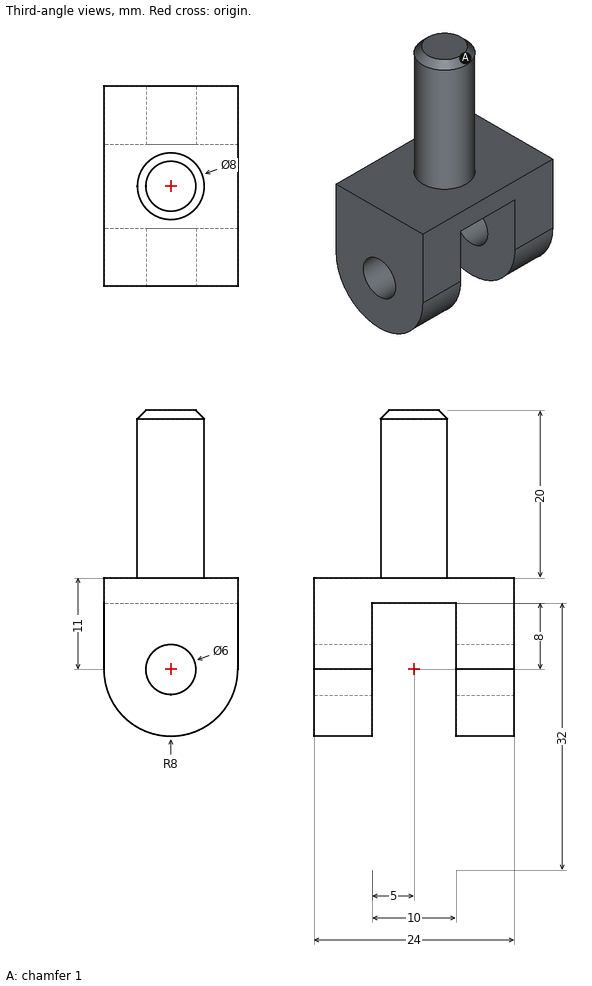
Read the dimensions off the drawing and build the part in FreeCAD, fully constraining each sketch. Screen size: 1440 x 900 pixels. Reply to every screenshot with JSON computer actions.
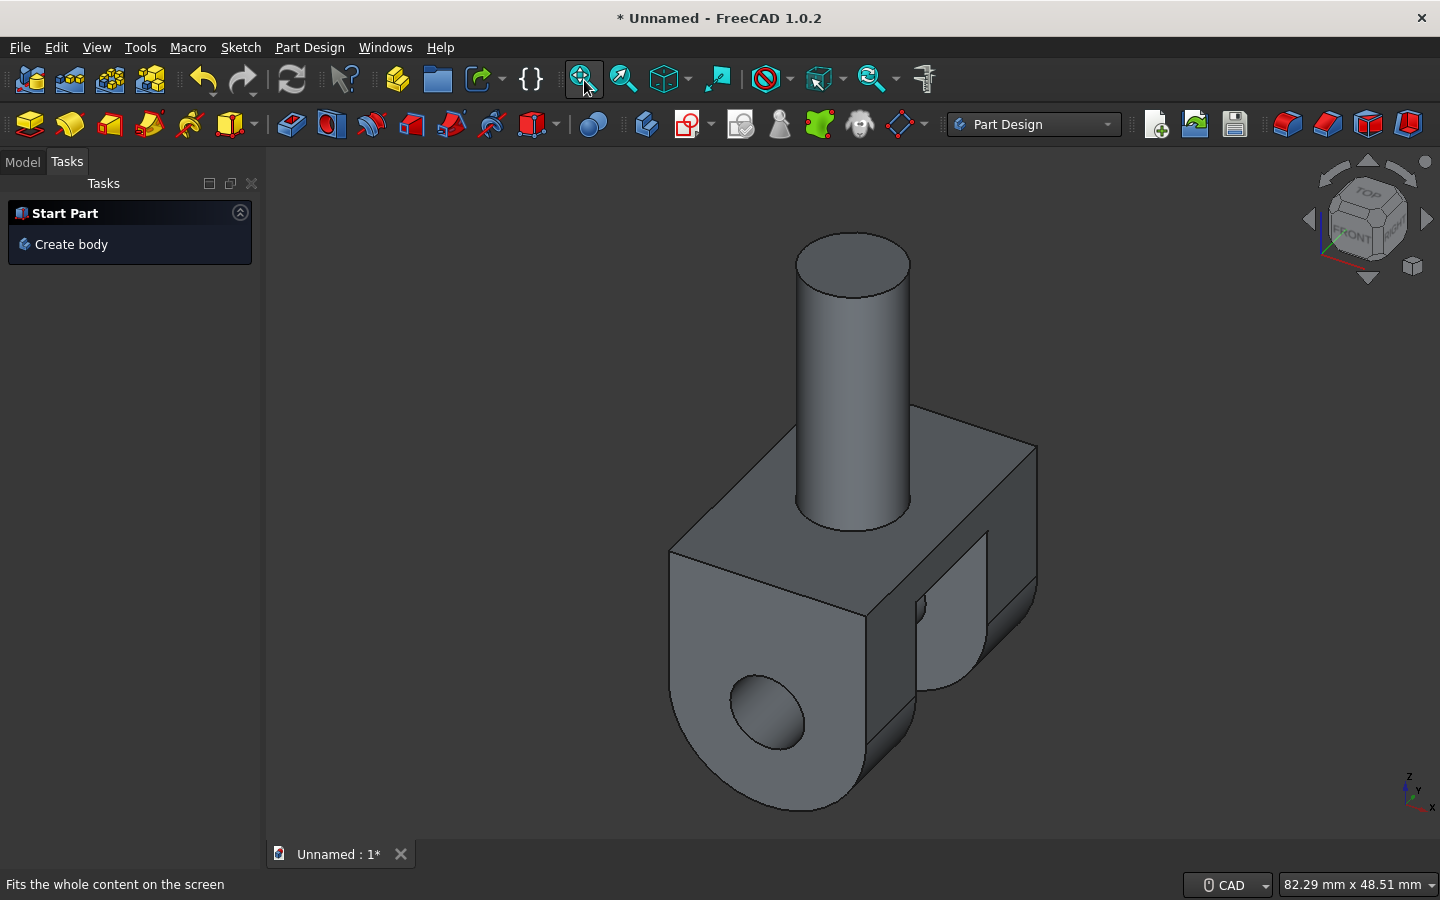
{"action": "left_click", "coordinate": [902, 280]}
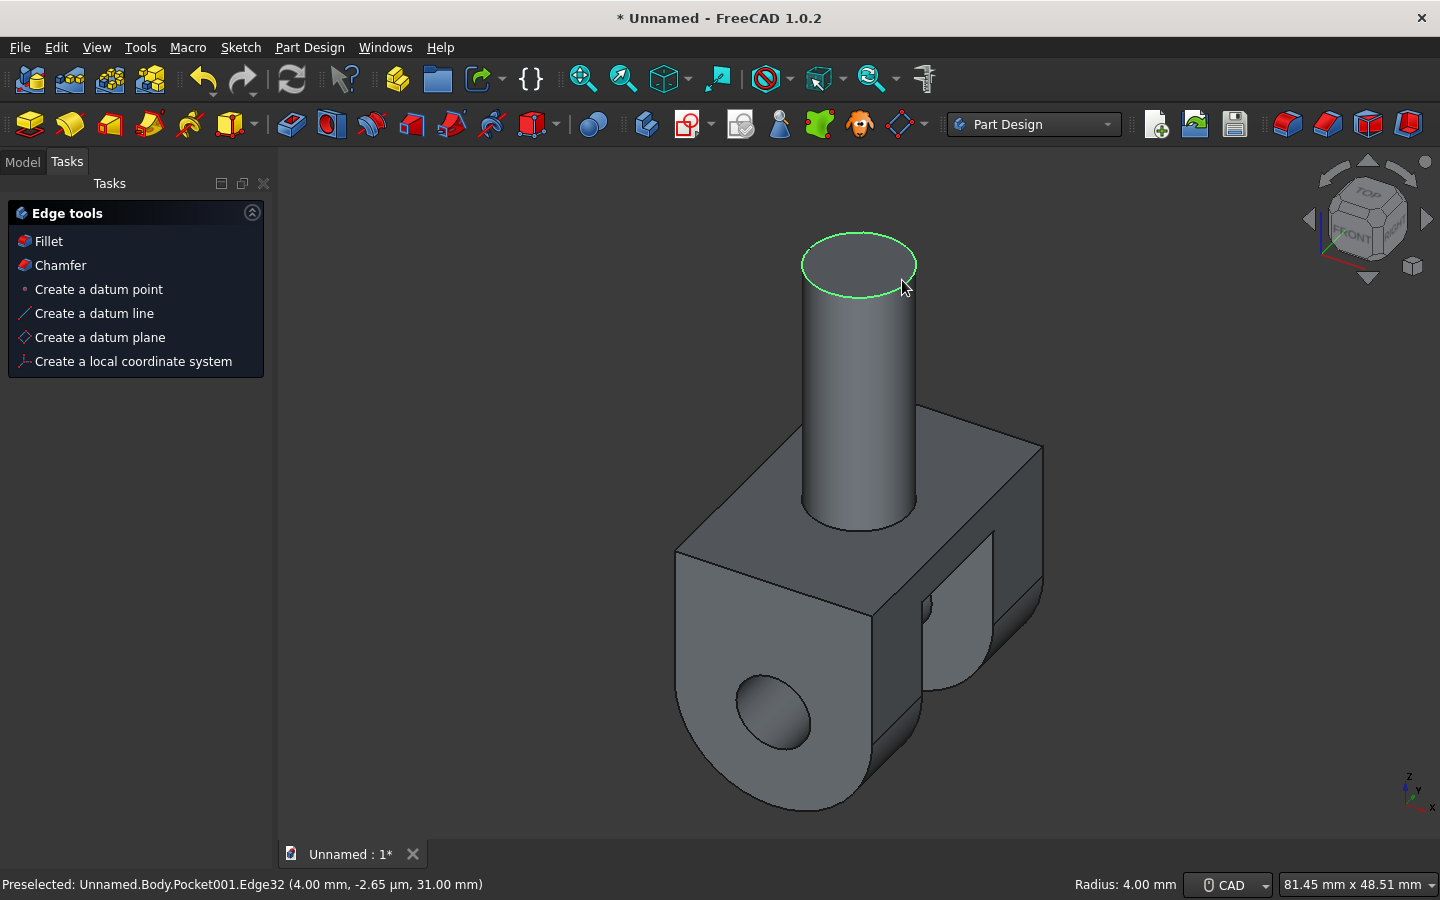
{"action": "left_click", "coordinate": [1328, 124]}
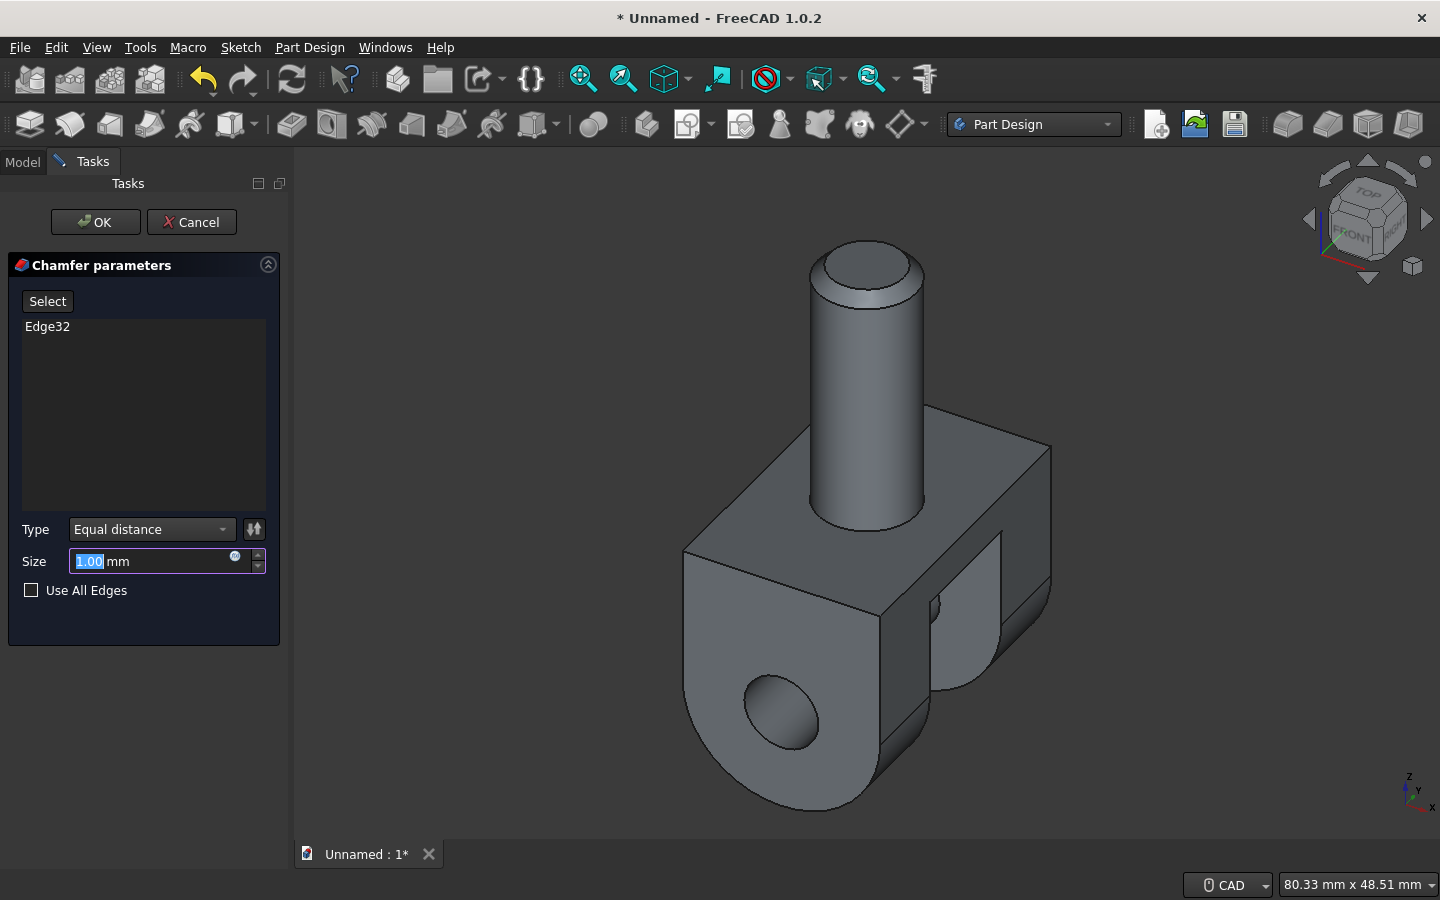
{"action": "type", "text": "1"}
{"action": "key", "text": "Tab"}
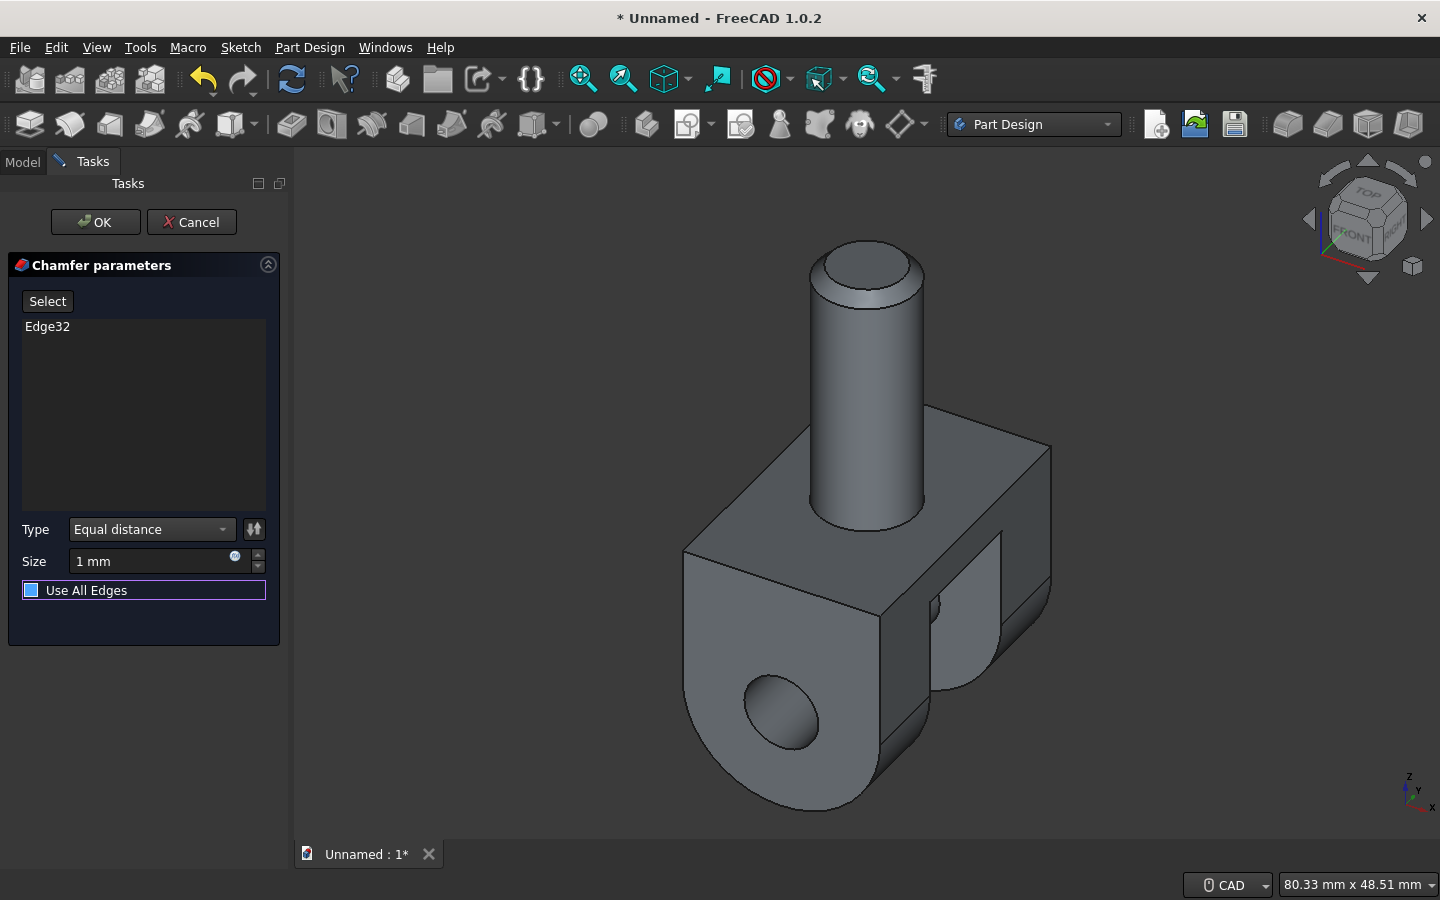
{"action": "left_click", "coordinate": [96, 222]}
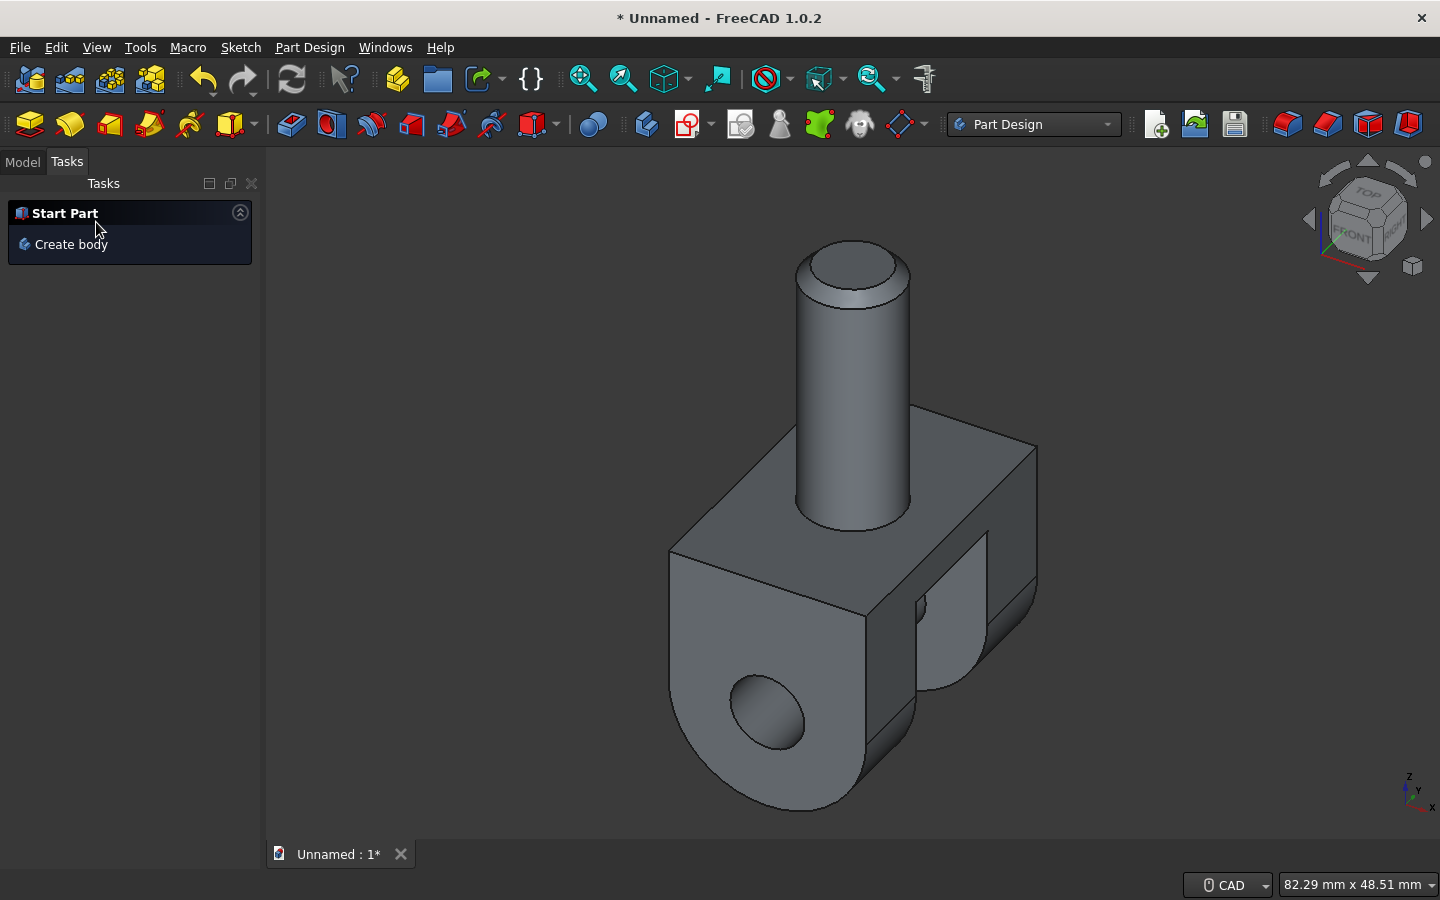
{"action": "key", "text": "0"}